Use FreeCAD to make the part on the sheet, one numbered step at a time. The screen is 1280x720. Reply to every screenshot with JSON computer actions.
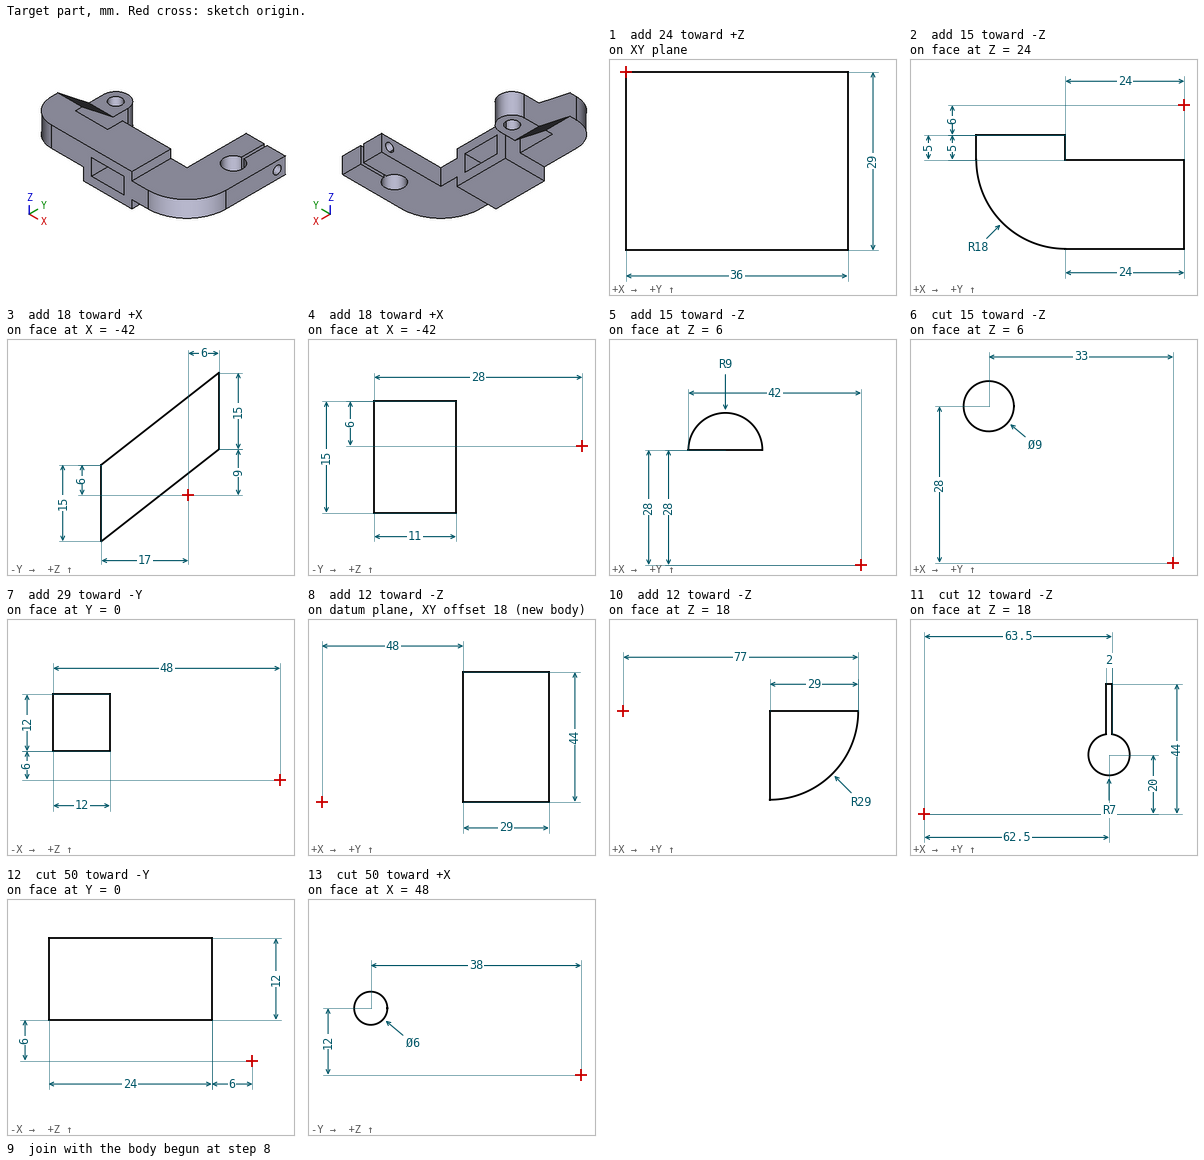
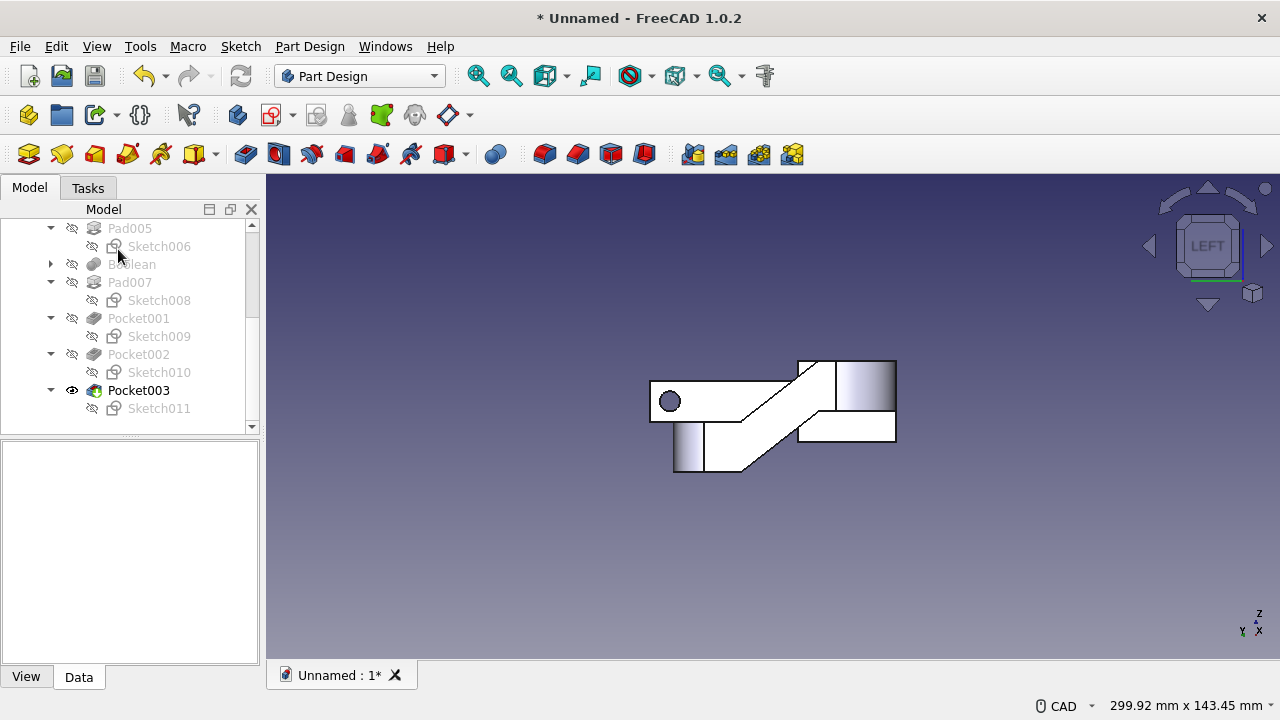
{"action": "key", "text": "0"}